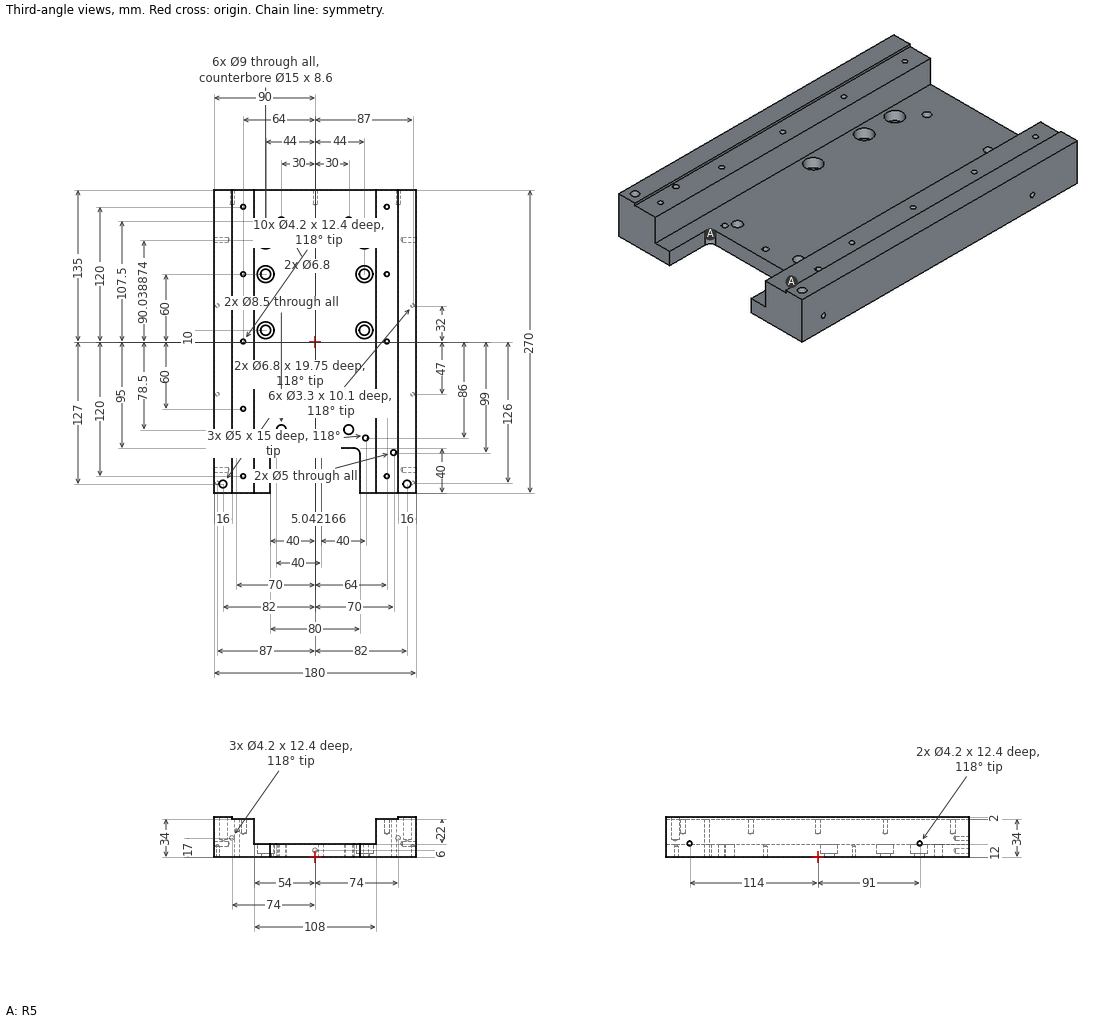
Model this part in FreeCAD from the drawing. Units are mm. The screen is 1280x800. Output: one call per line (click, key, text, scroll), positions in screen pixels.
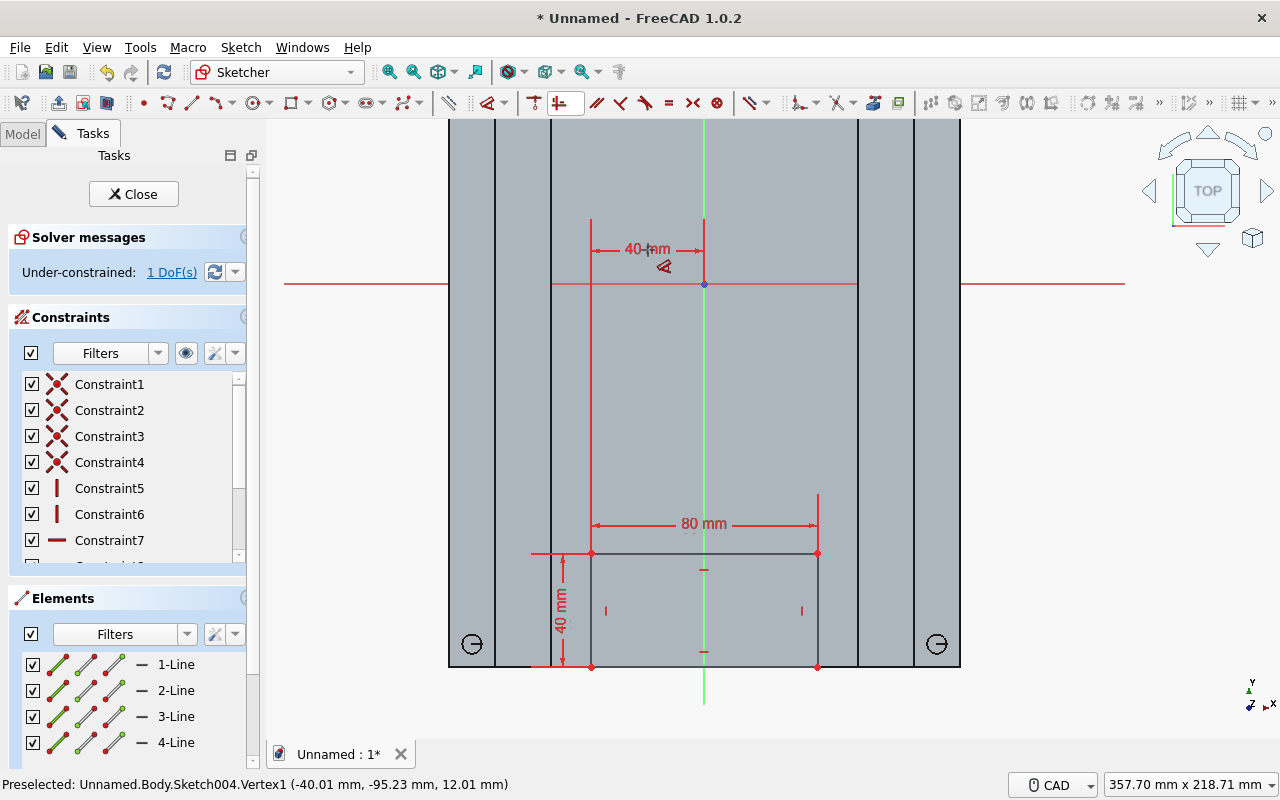
click(591, 554)
click(557, 419)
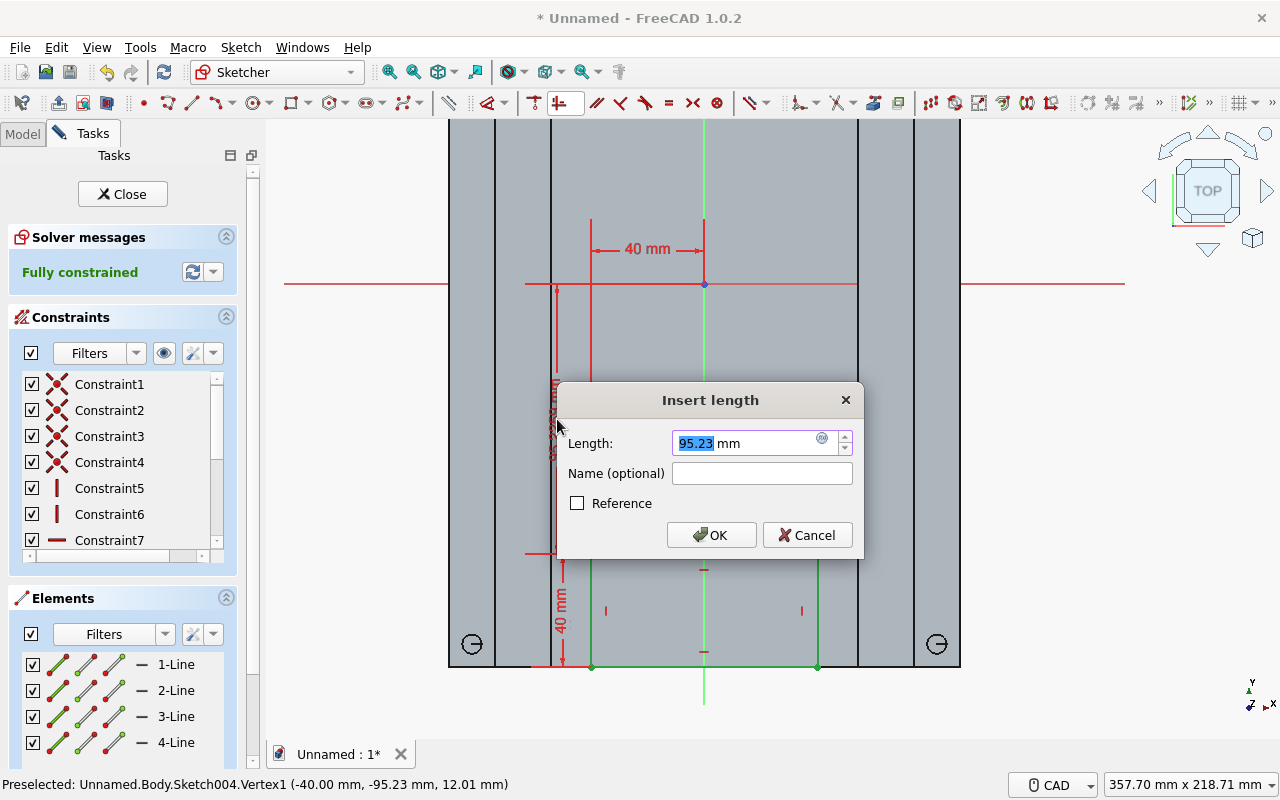
text(95)
key(Return)
key(Escape)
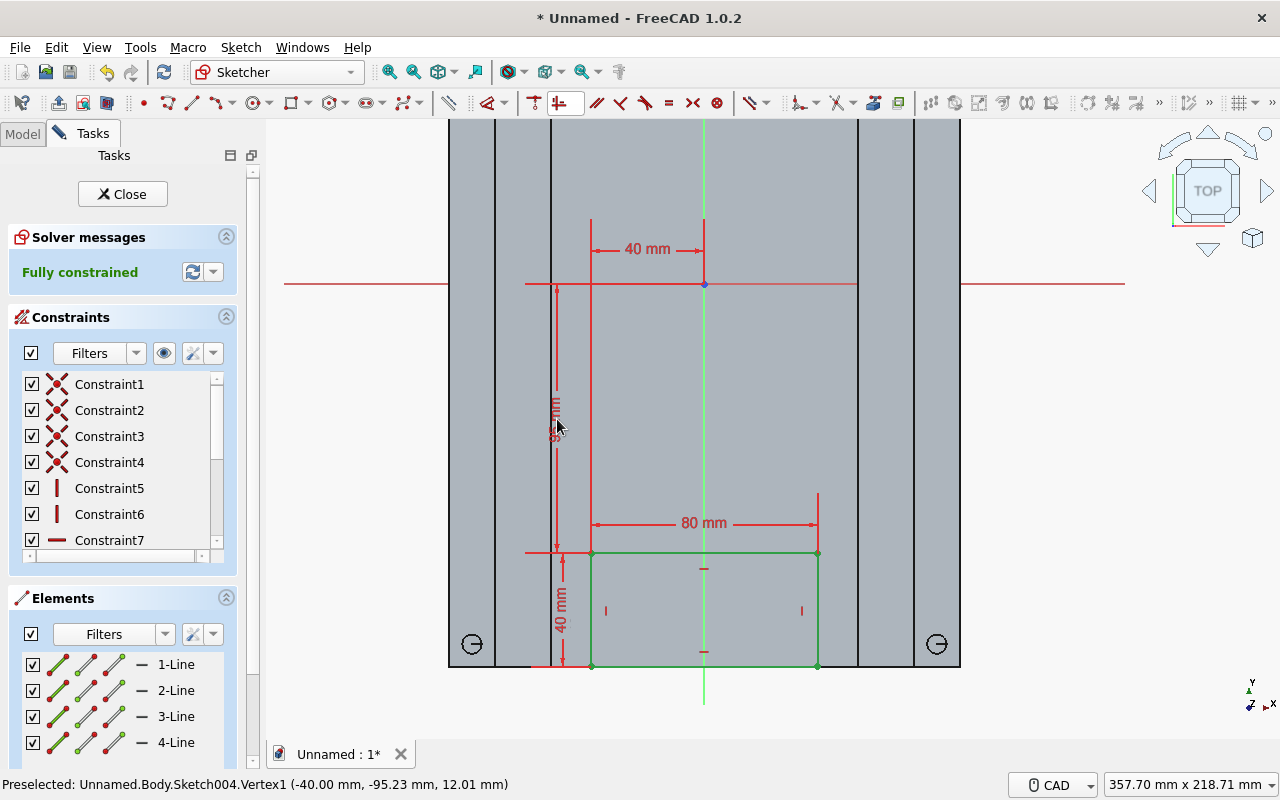
click(123, 194)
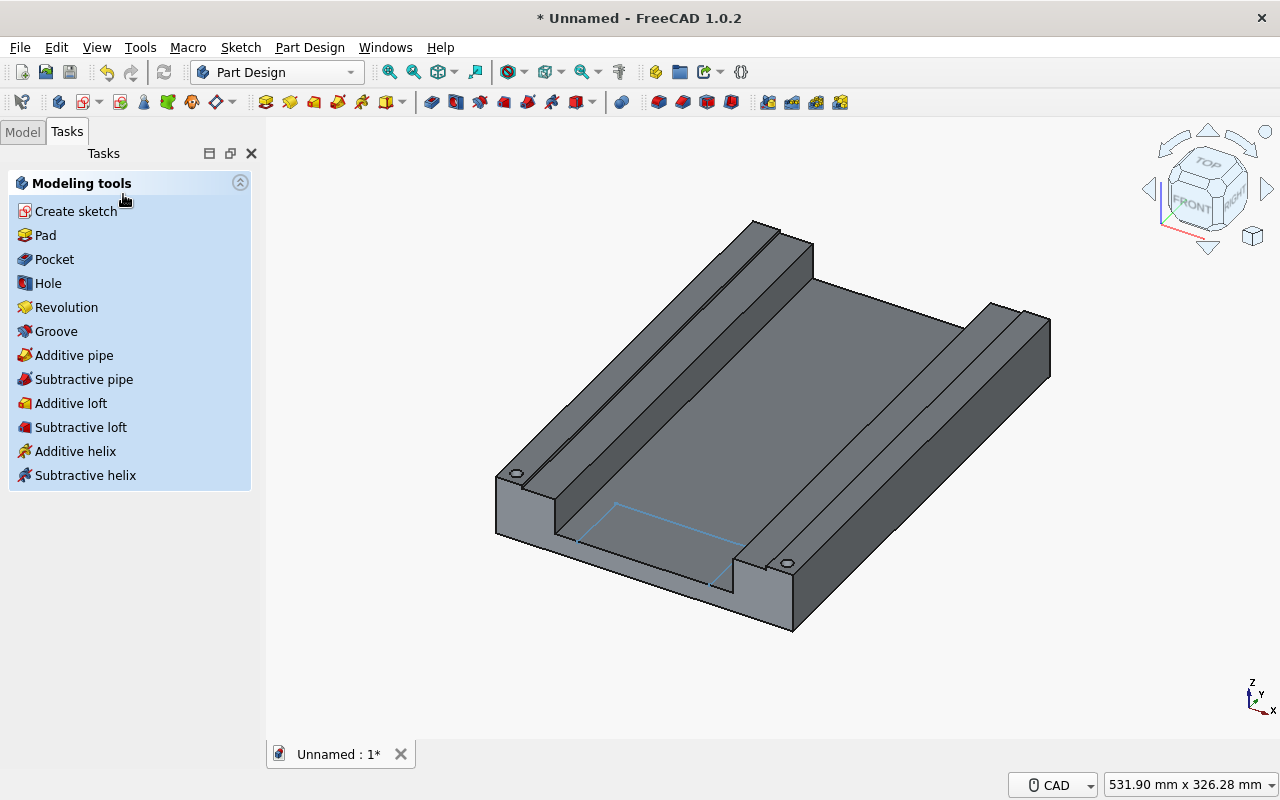
click(432, 102)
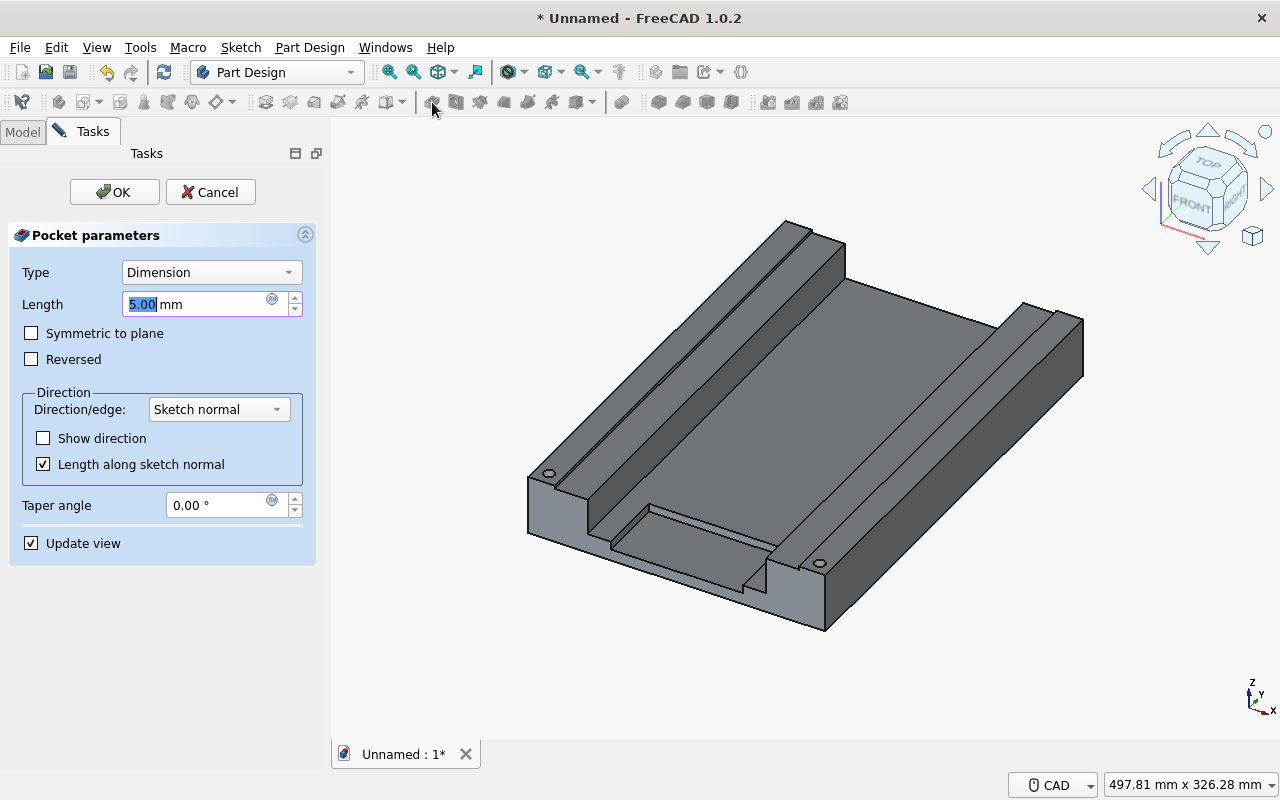
click(212, 272)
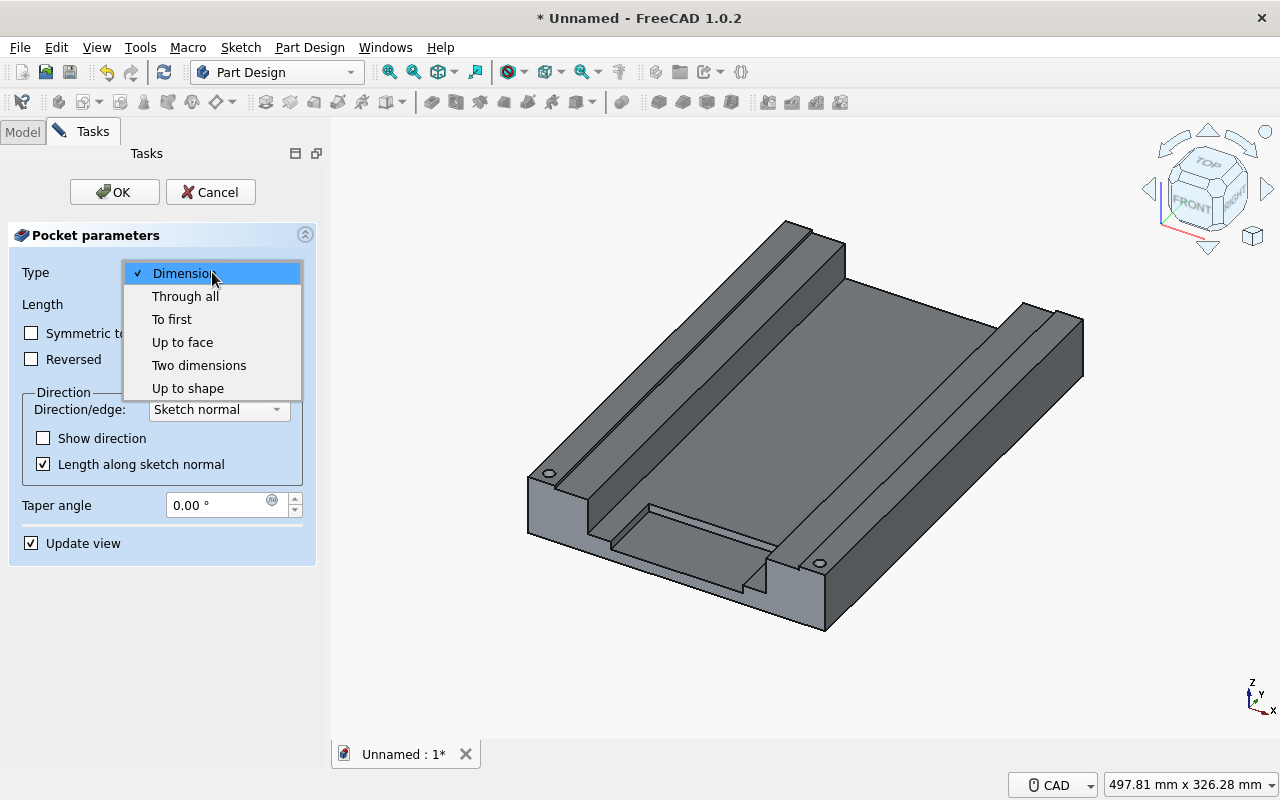
click(212, 296)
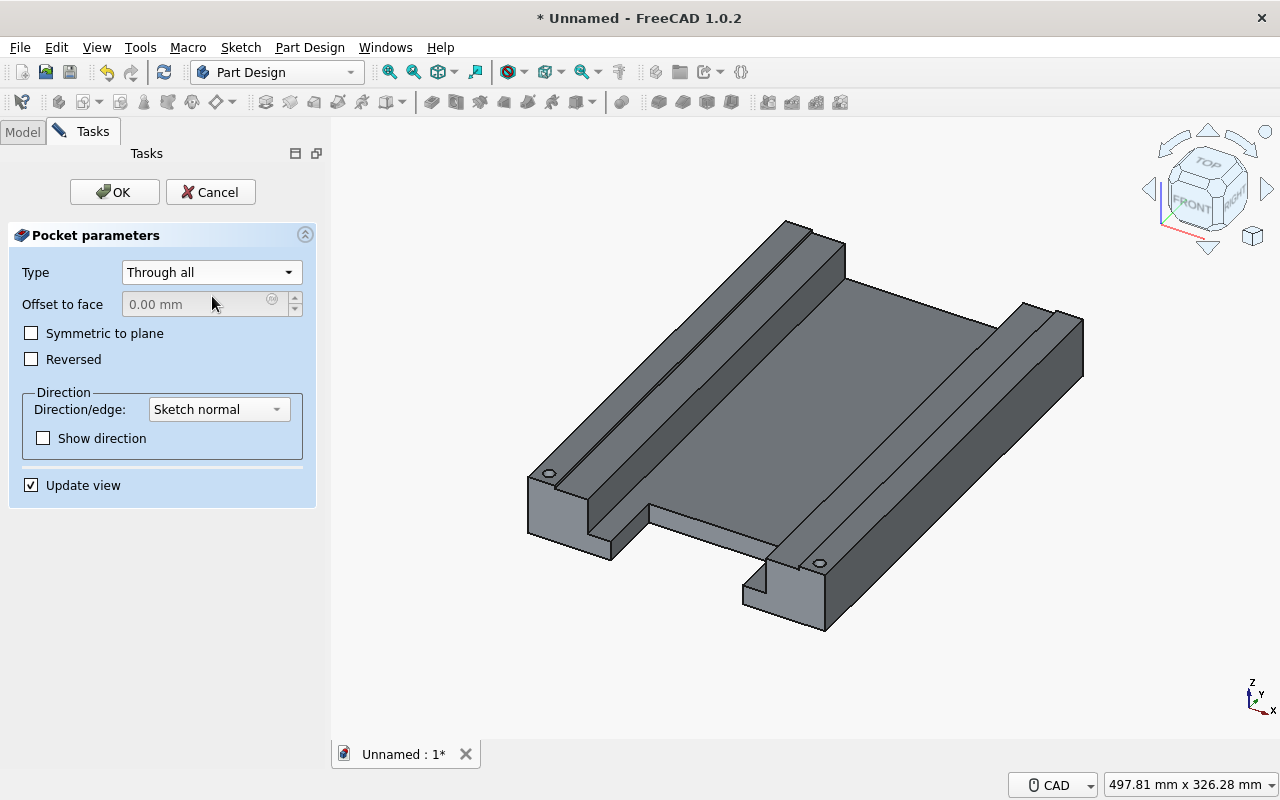
click(115, 192)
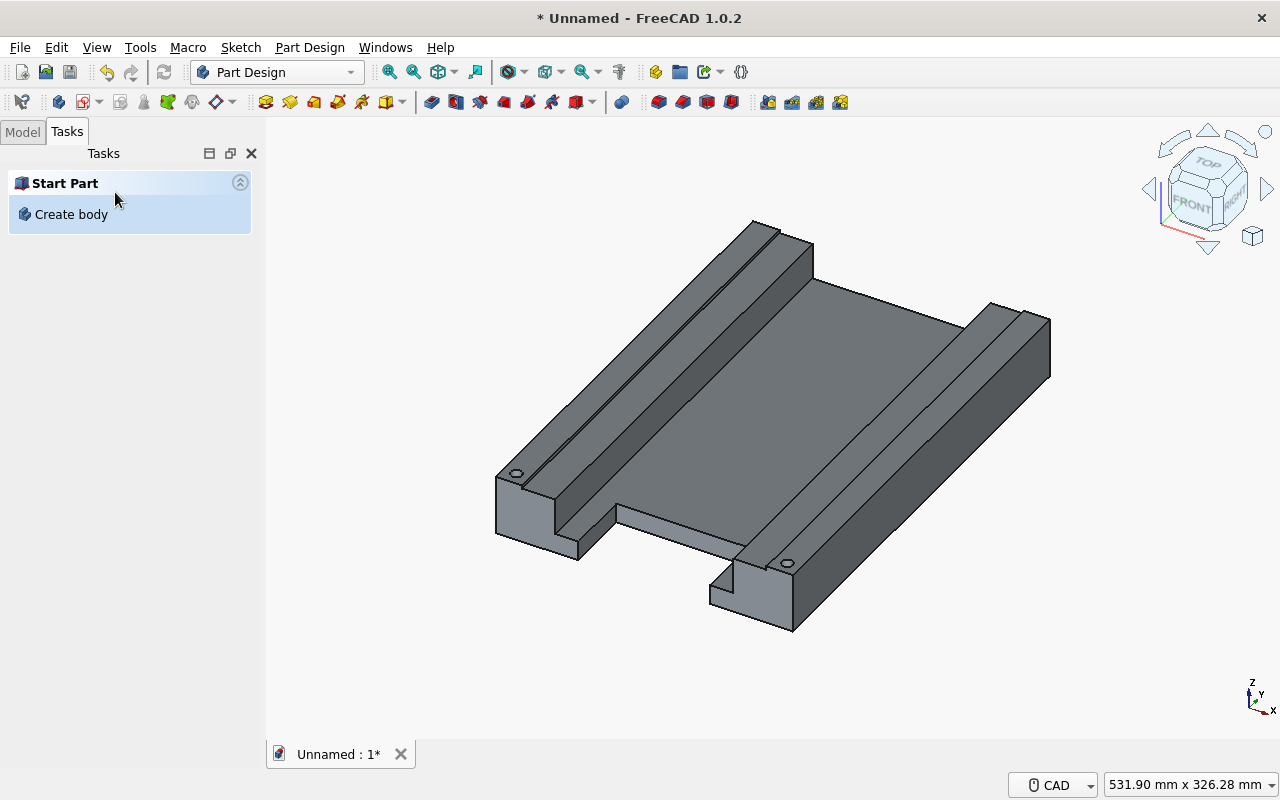
key(0)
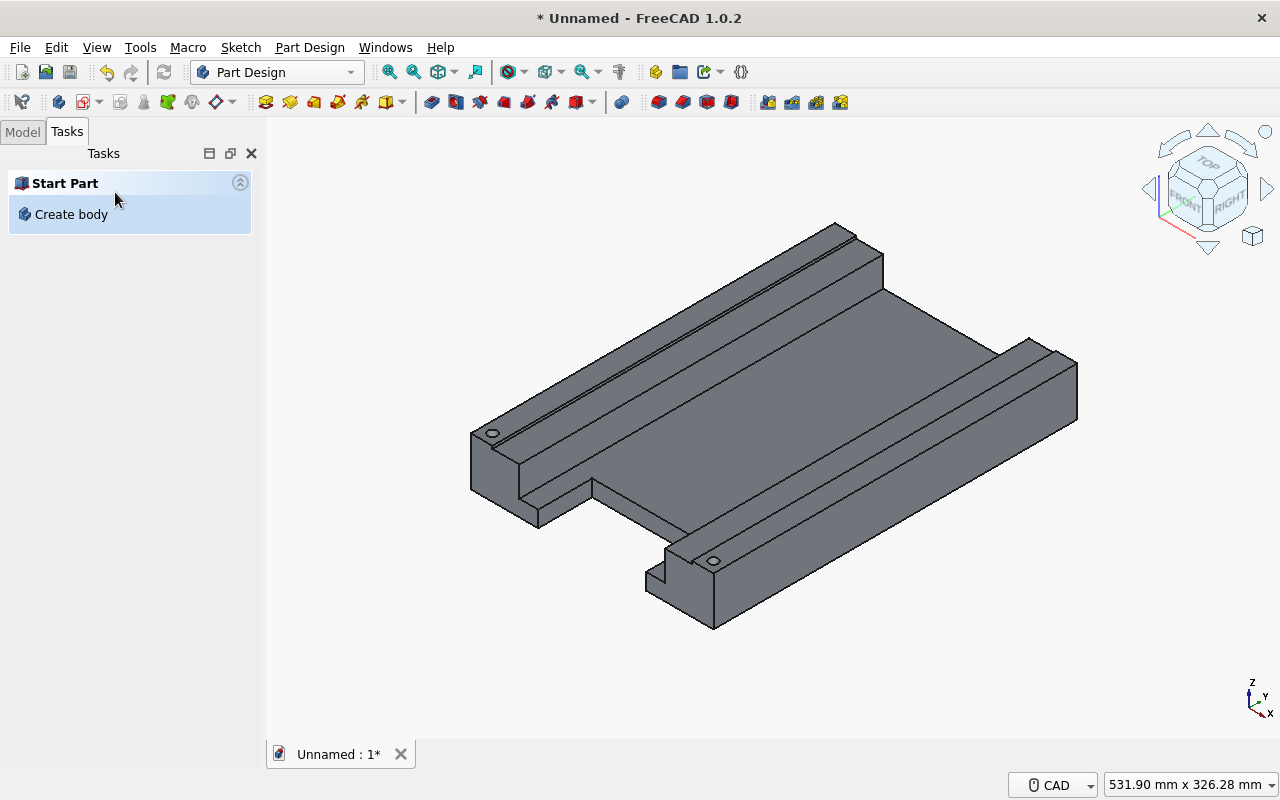
key(2)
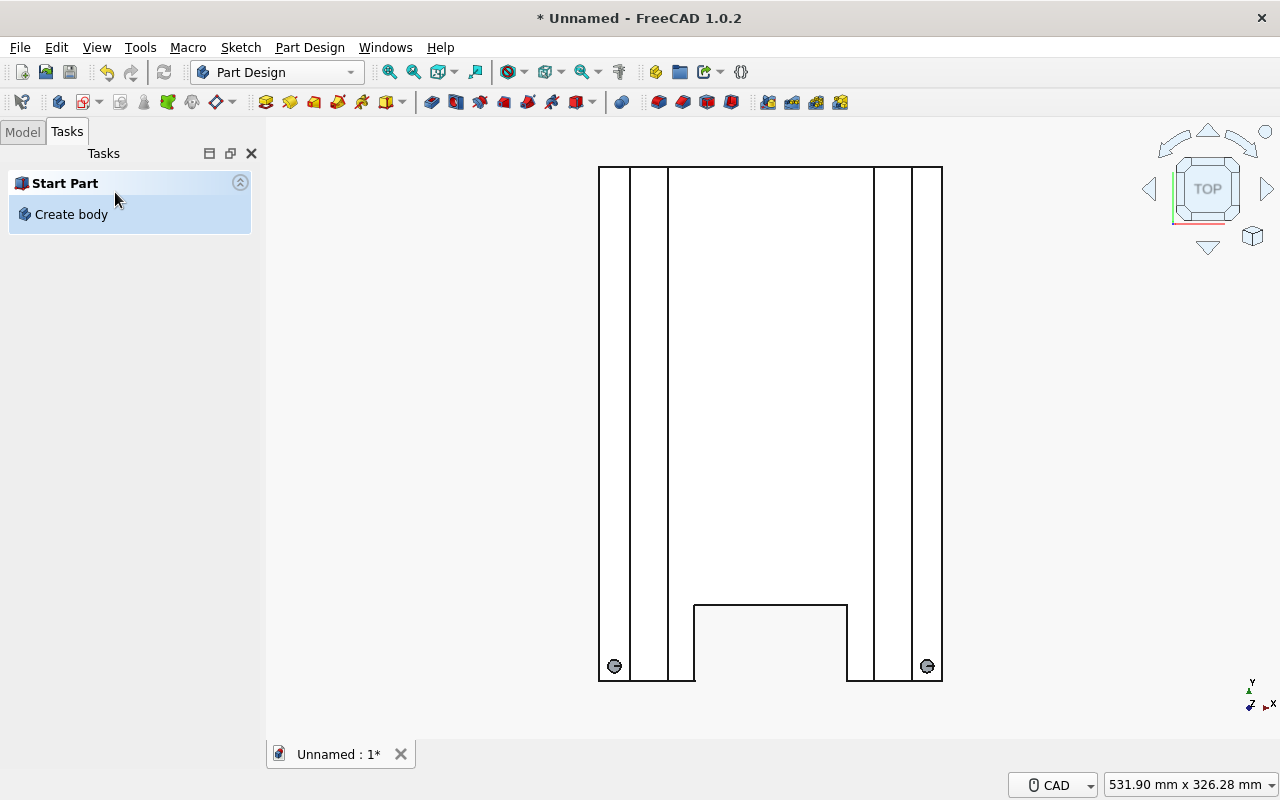
key(1)